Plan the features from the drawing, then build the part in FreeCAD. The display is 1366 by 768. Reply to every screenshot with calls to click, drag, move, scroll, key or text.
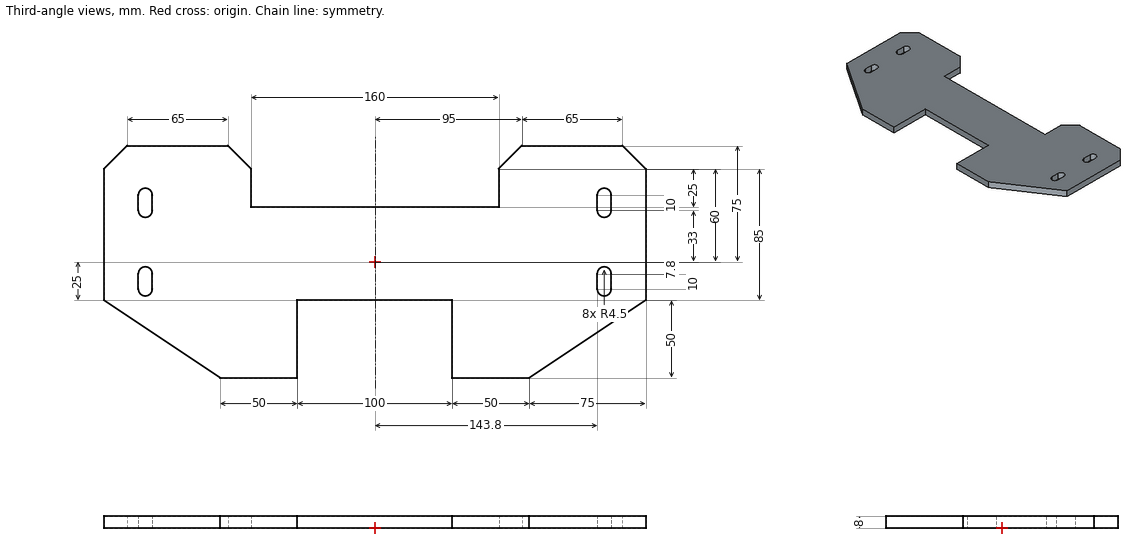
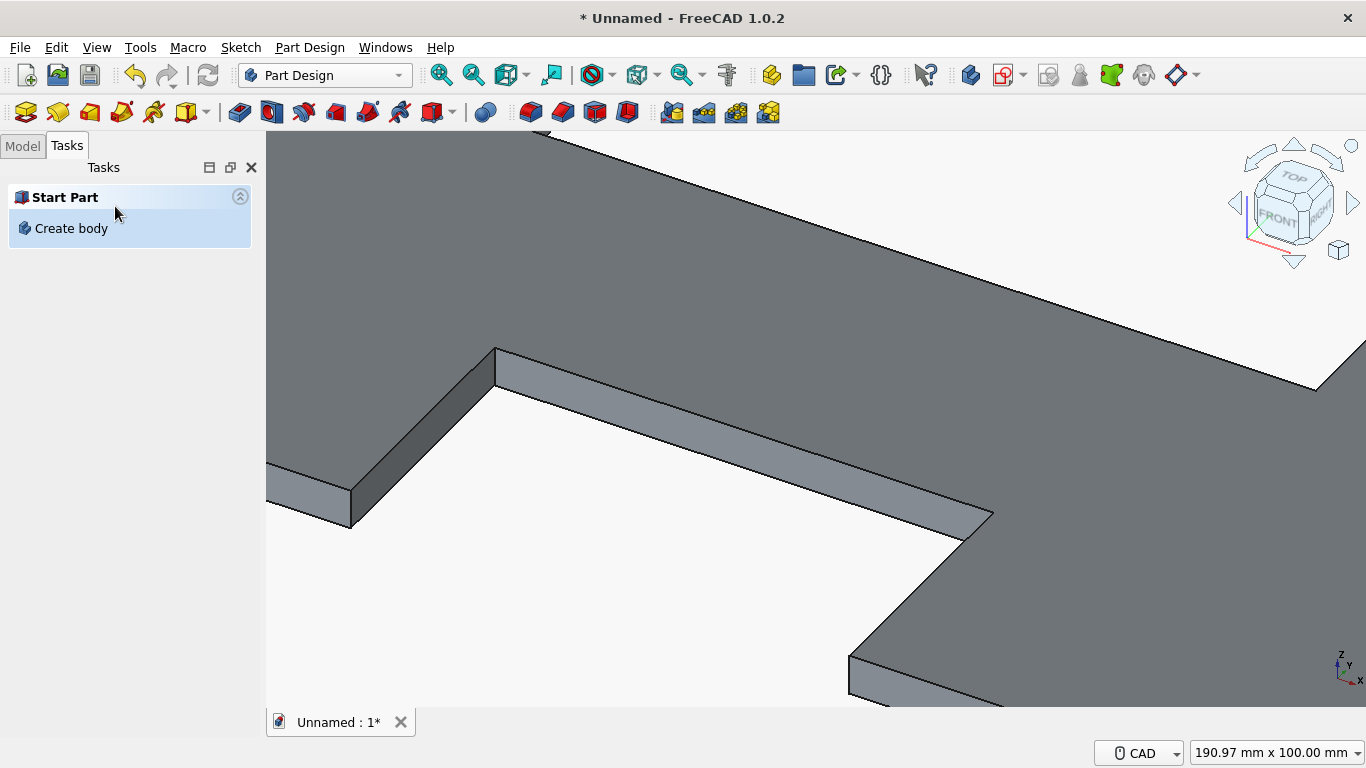
key(0)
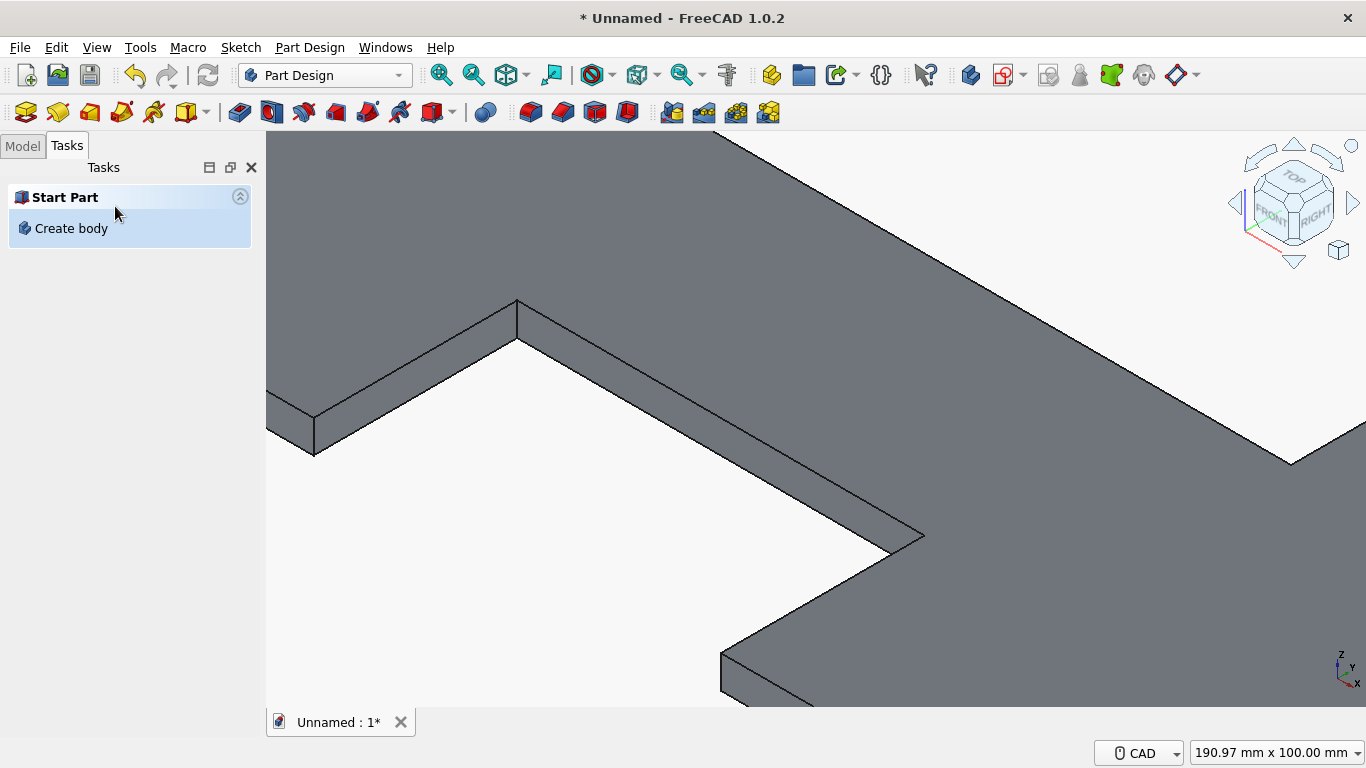
click(442, 76)